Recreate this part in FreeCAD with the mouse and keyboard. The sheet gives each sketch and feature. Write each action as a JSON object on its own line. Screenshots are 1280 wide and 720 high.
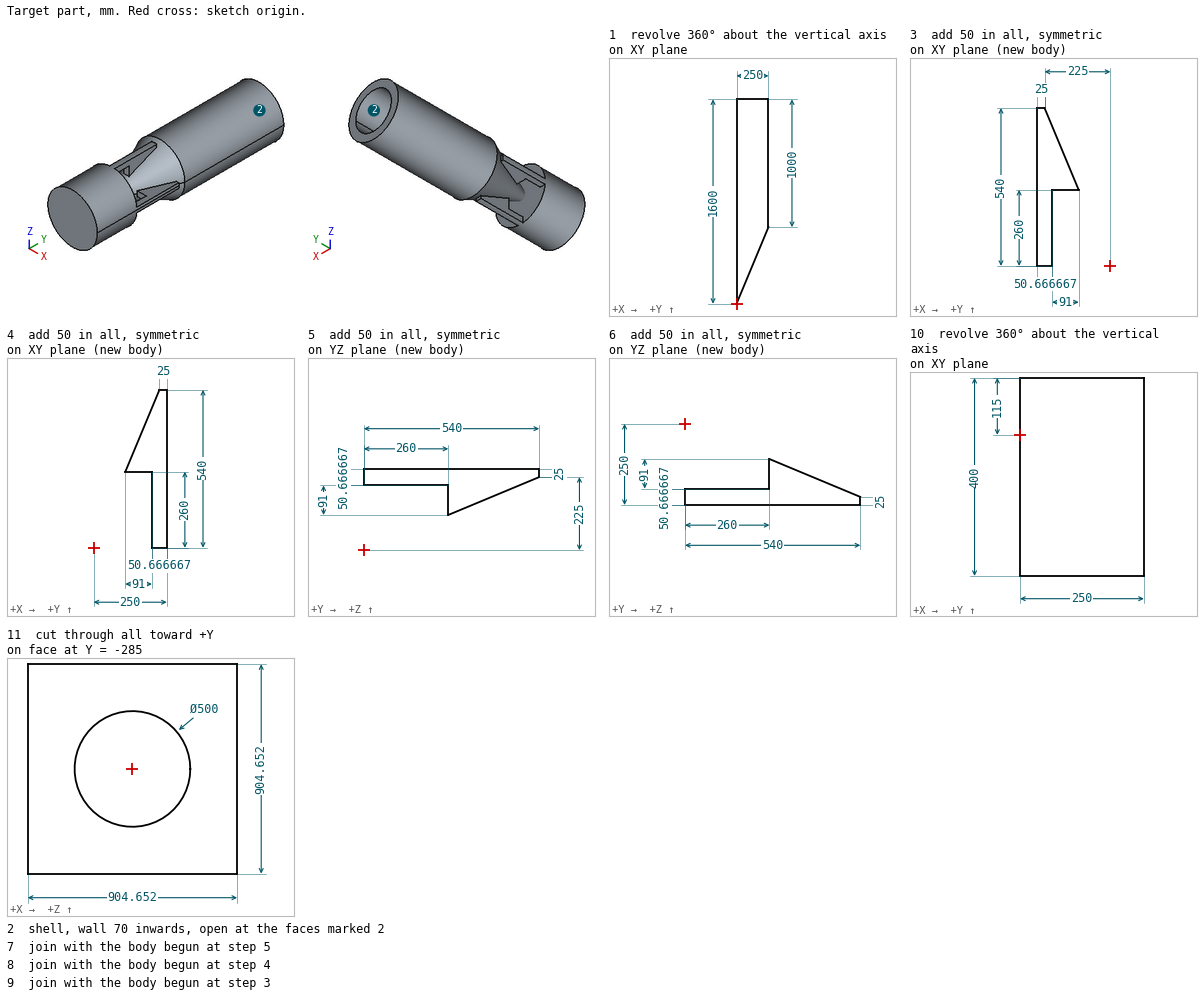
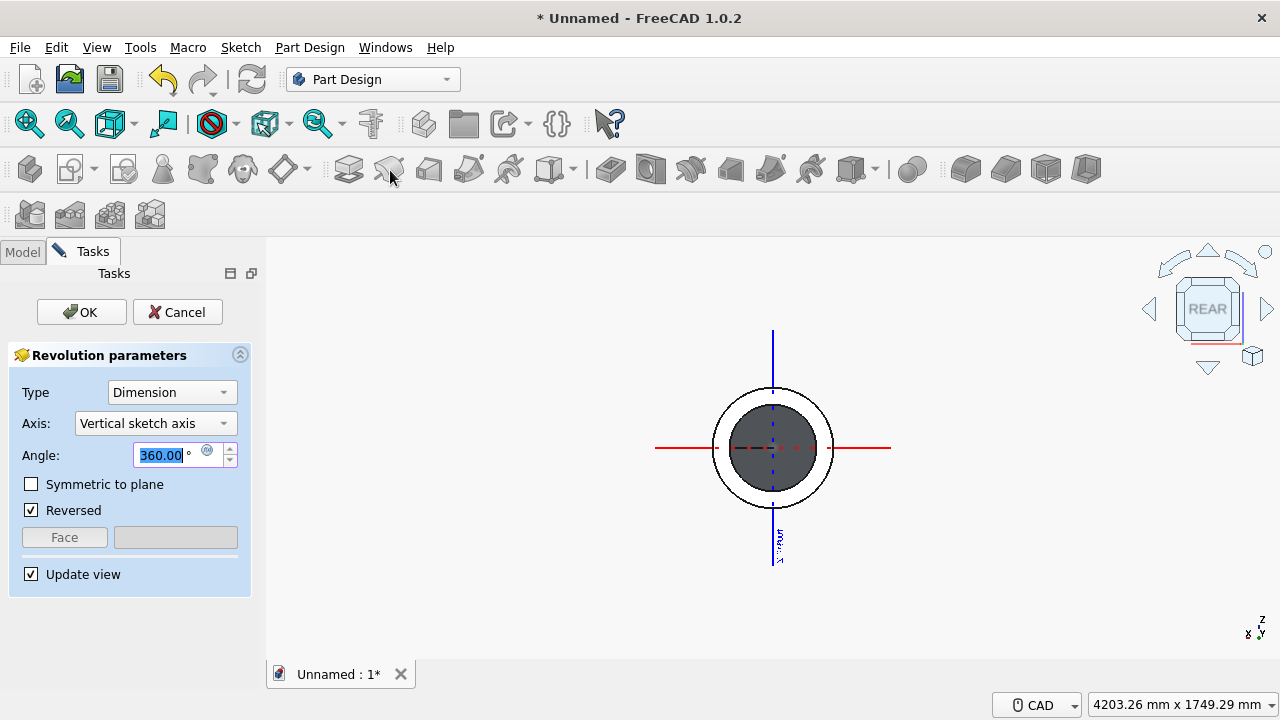
{"action": "left_click", "coordinate": [82, 312]}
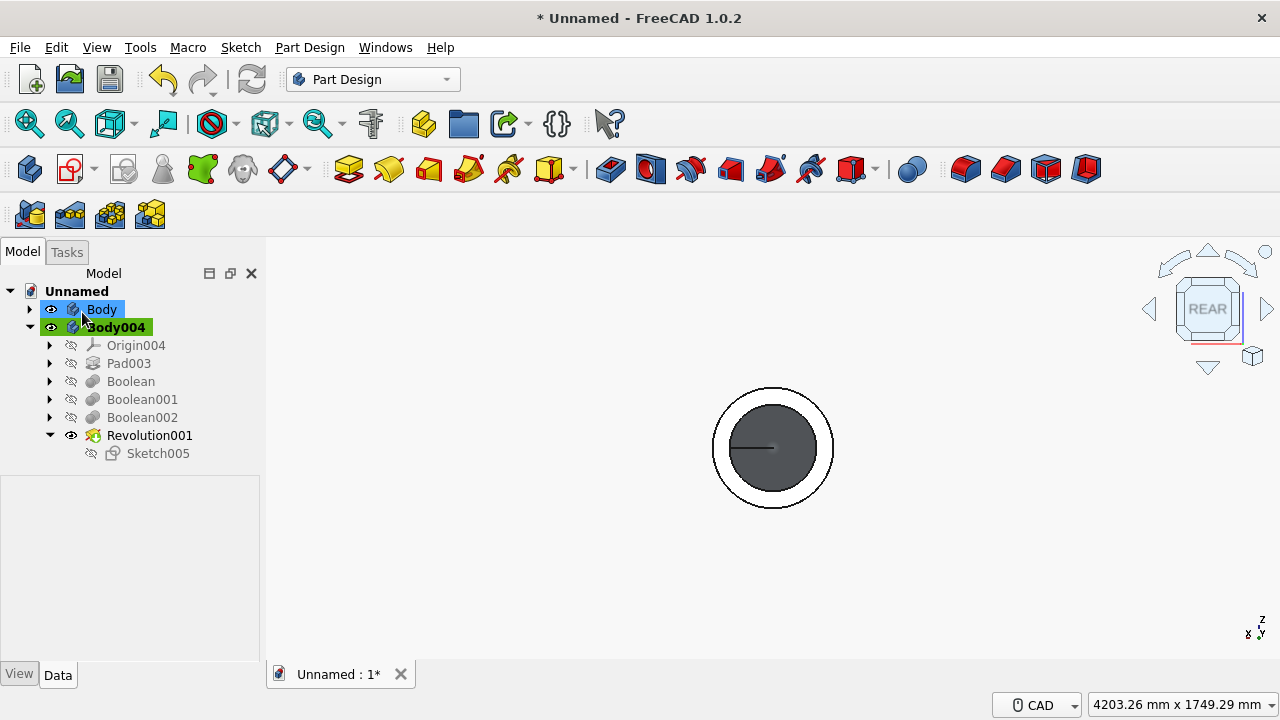
{"action": "left_click", "coordinate": [30, 124]}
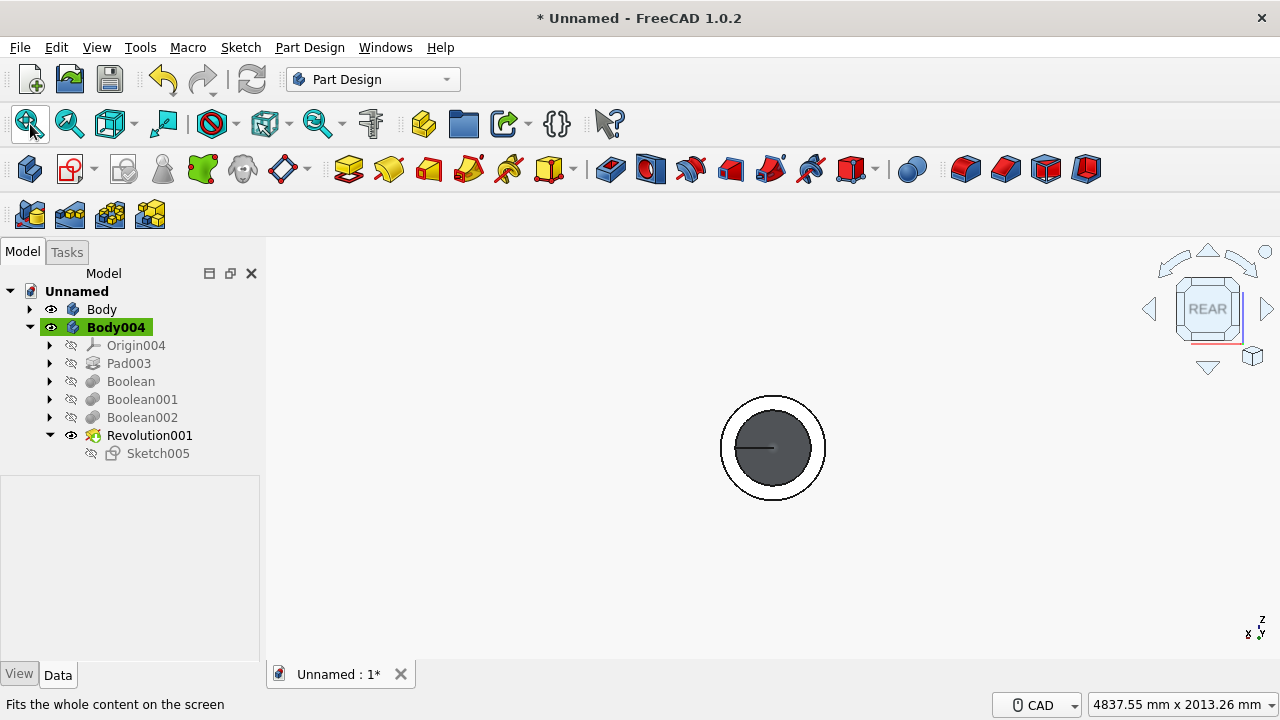
{"action": "key", "text": "0"}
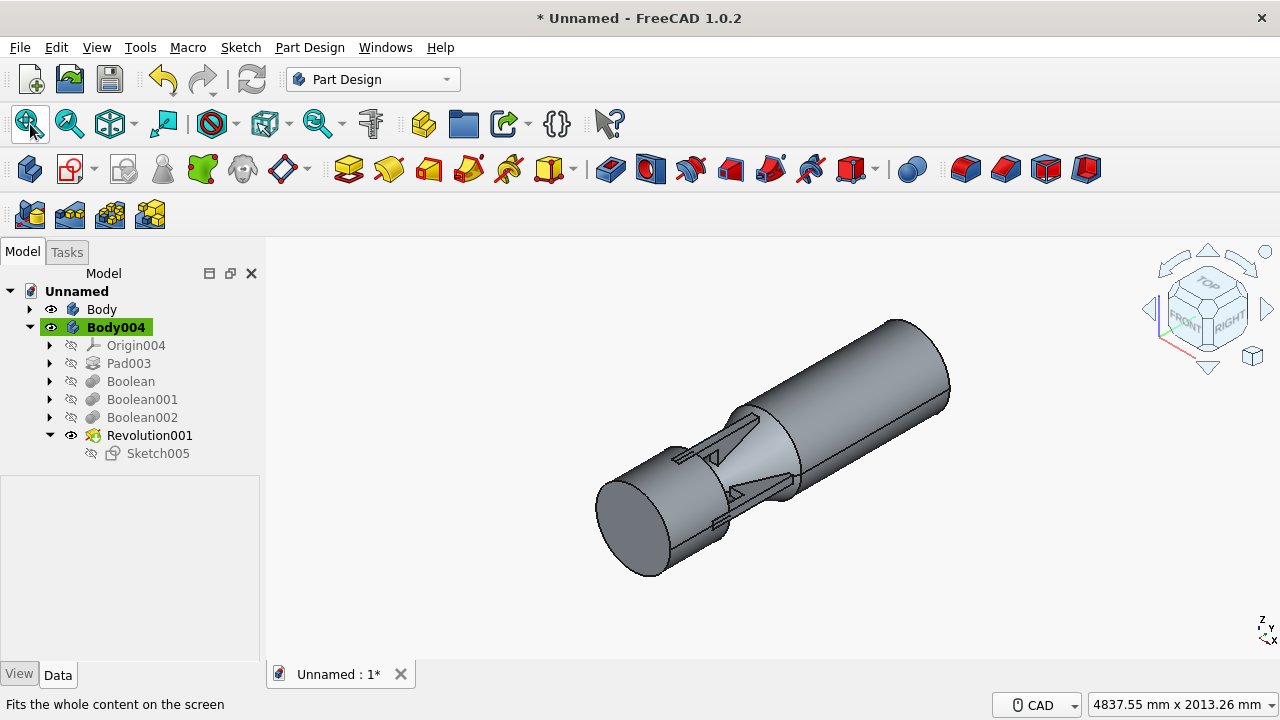
{"action": "left_click", "coordinate": [633, 528]}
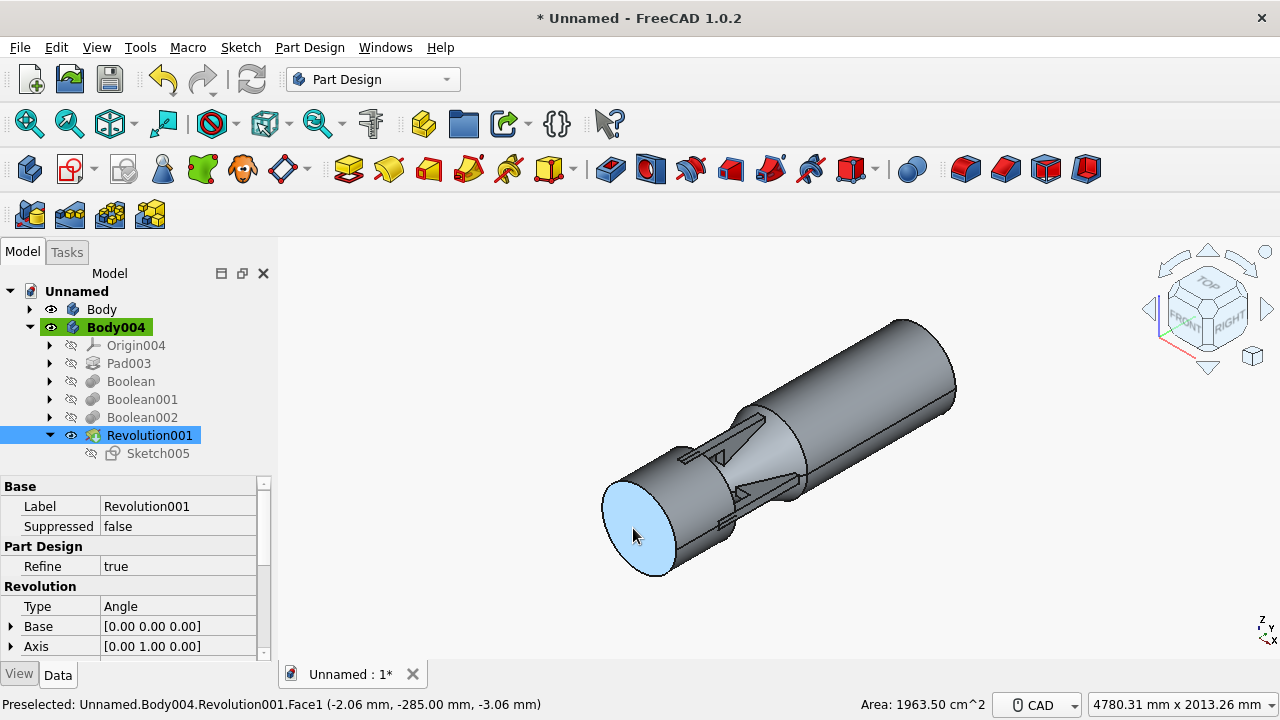
{"action": "left_click", "coordinate": [70, 170]}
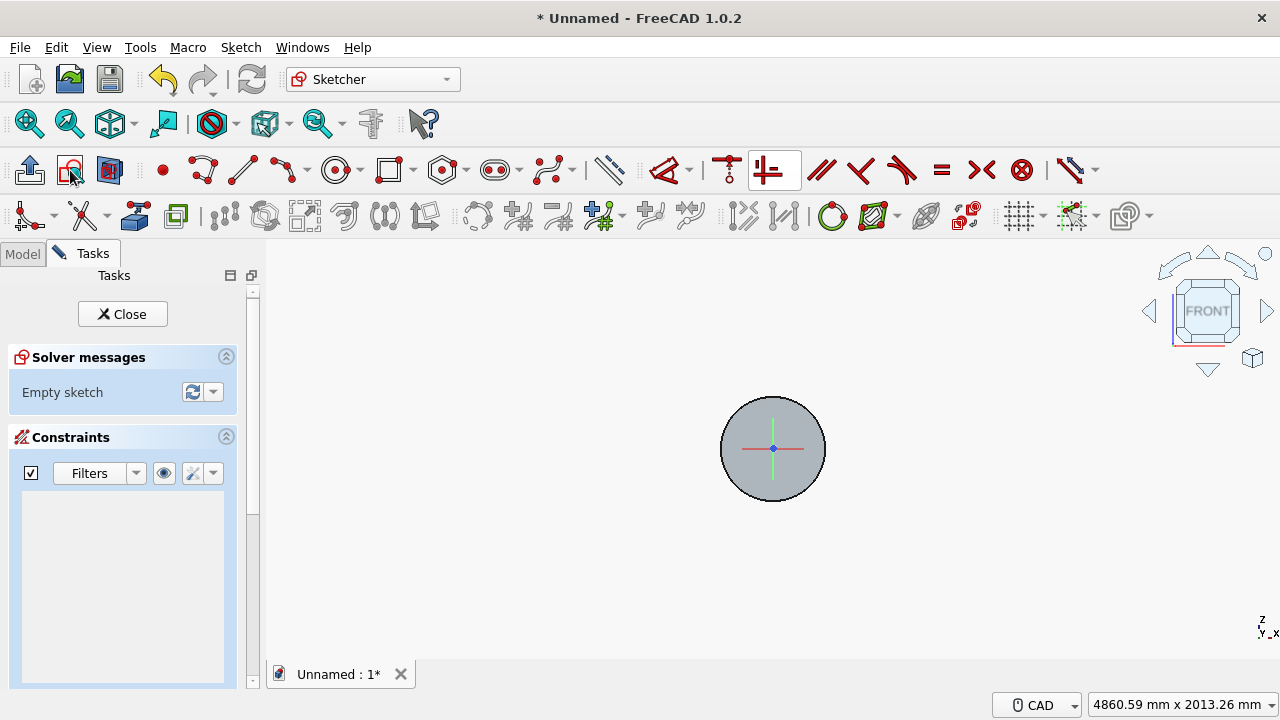
{"action": "scroll", "coordinate": [912, 449], "scroll_direction": "up", "scroll_amount": 2}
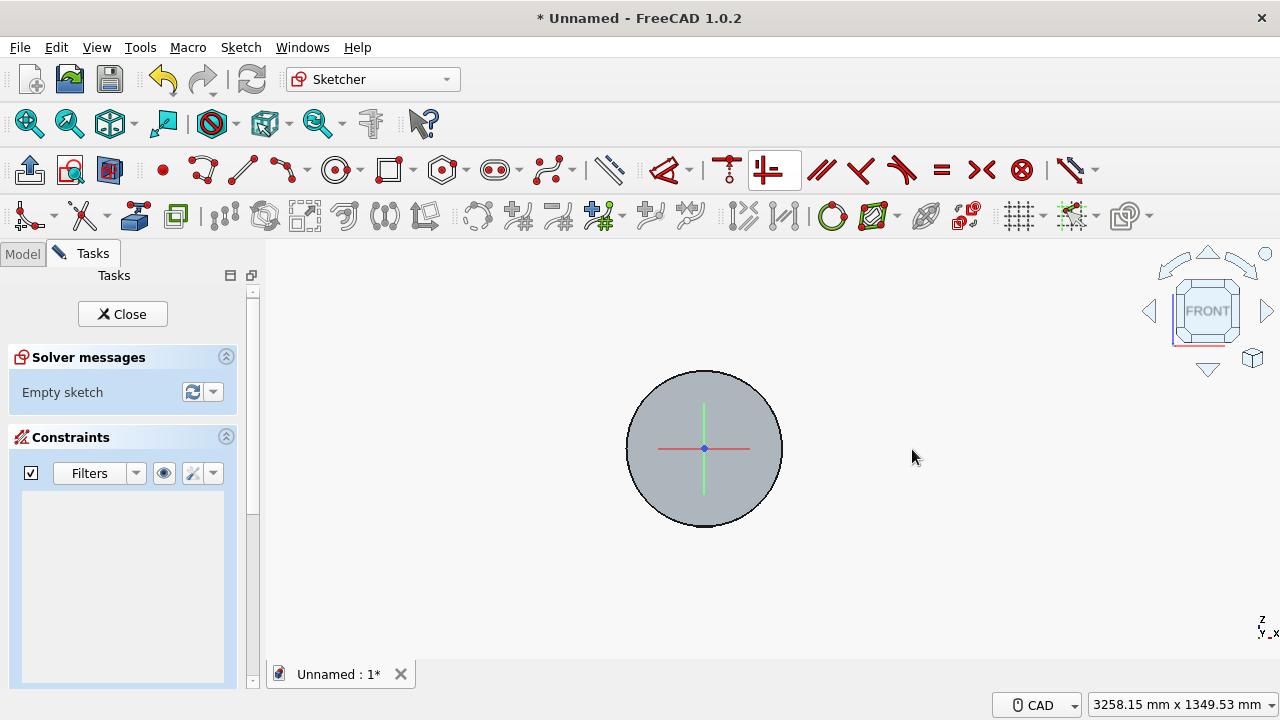
{"action": "key", "text": "g v"}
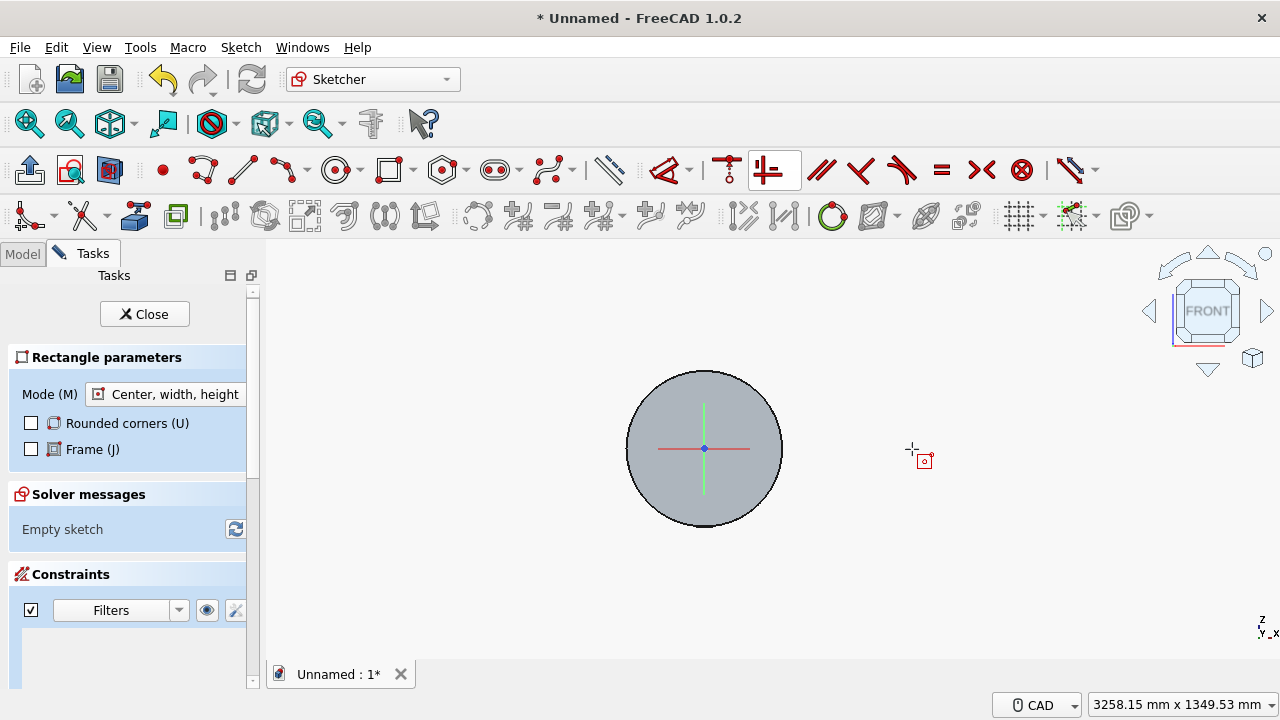
{"action": "left_click", "coordinate": [704, 449]}
{"action": "left_click", "coordinate": [845, 308]}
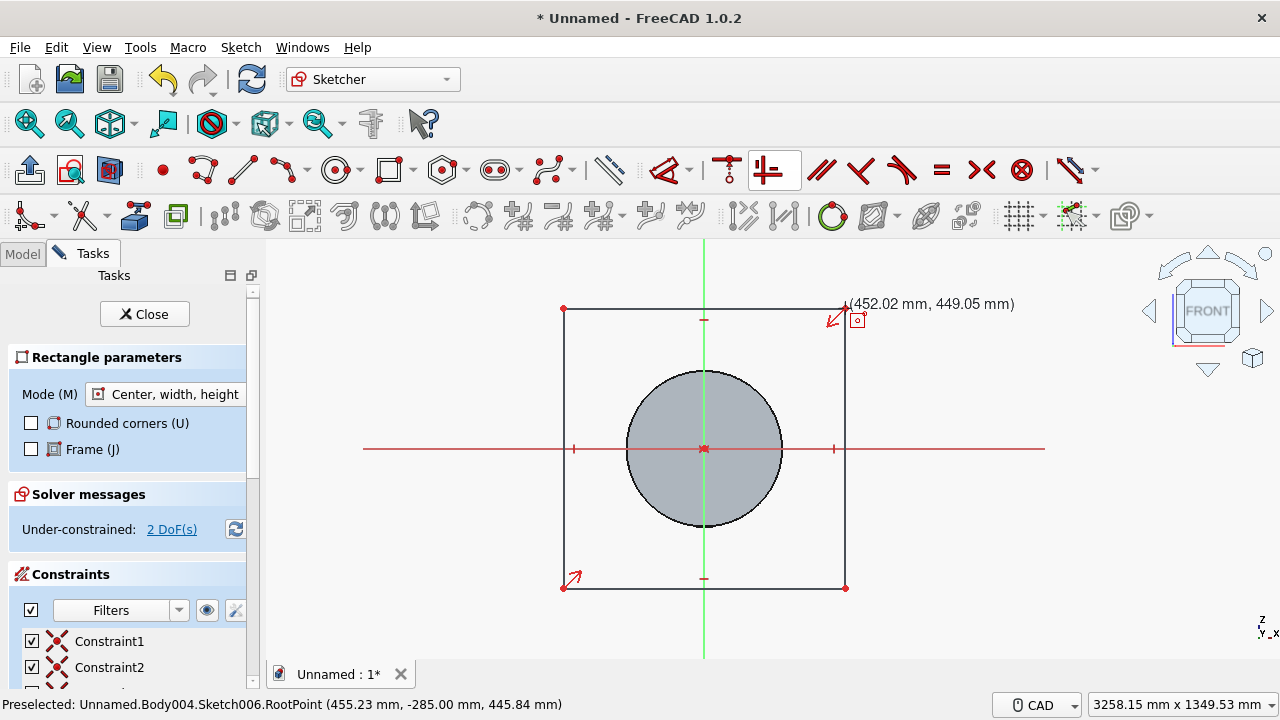
{"action": "left_click", "coordinate": [336, 170]}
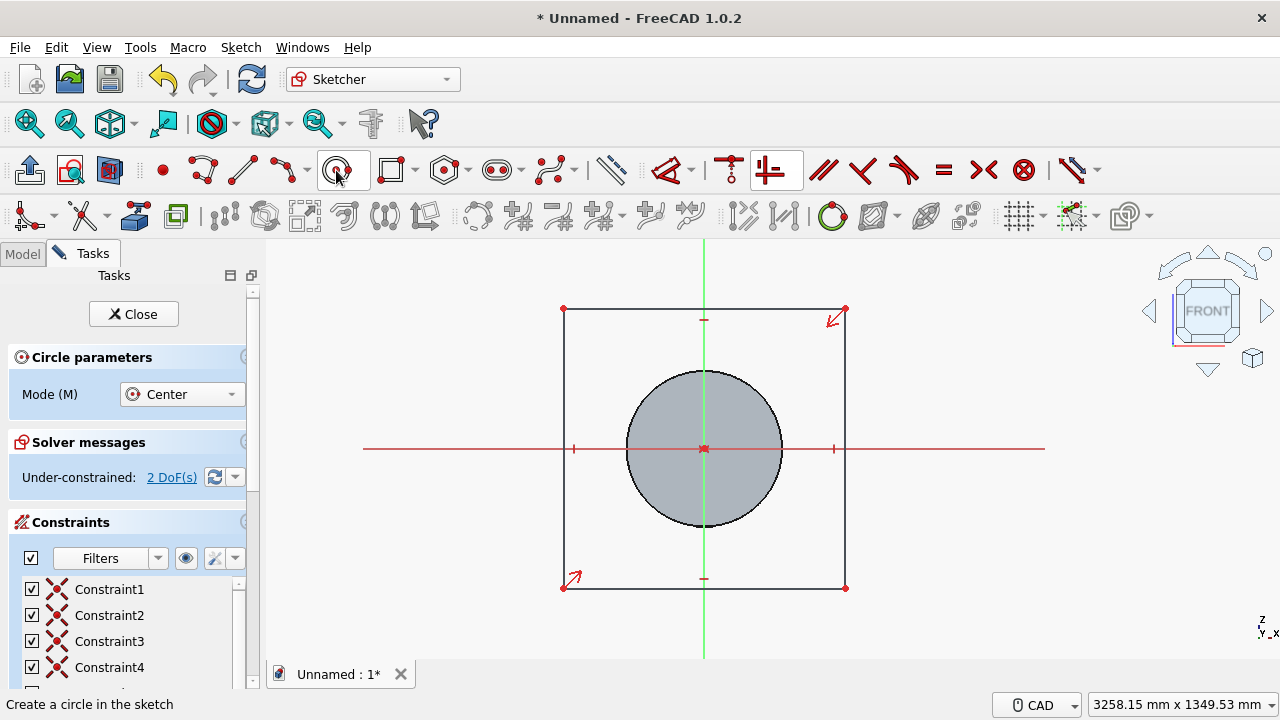
{"action": "left_click", "coordinate": [704, 449]}
{"action": "left_click", "coordinate": [759, 394]}
{"action": "key", "text": "Escape"}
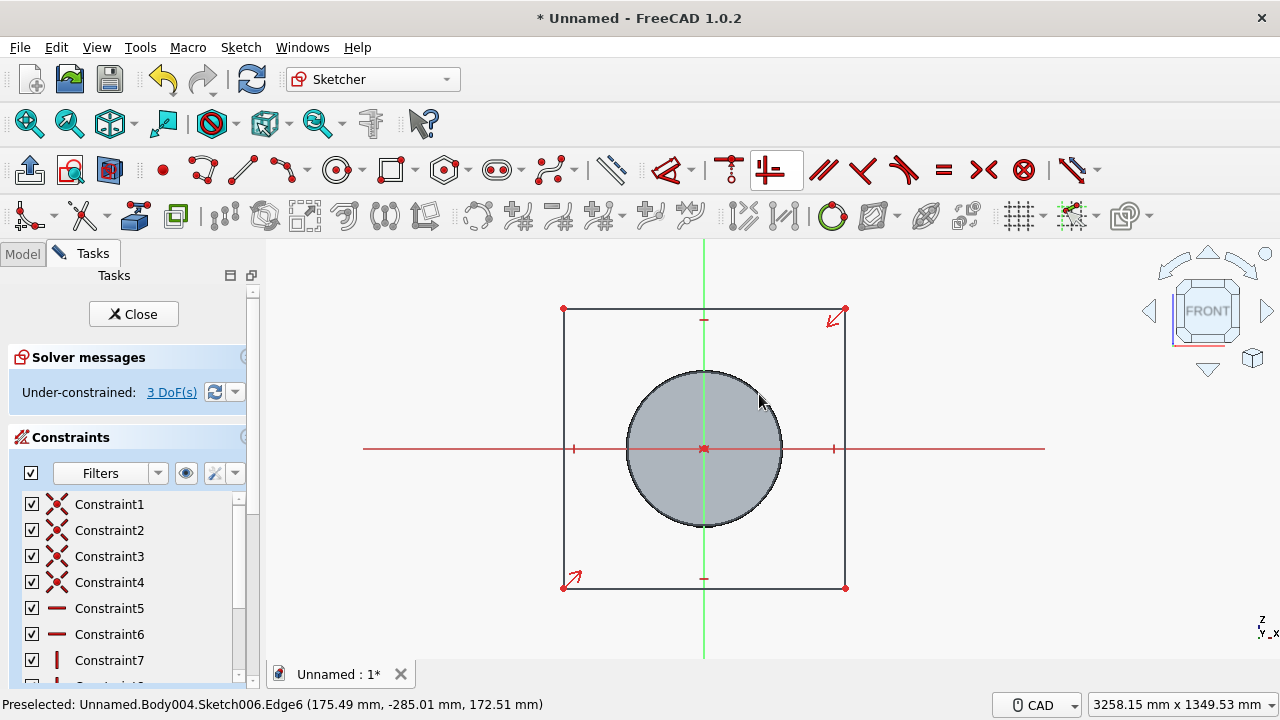
{"action": "left_click", "coordinate": [666, 170]}